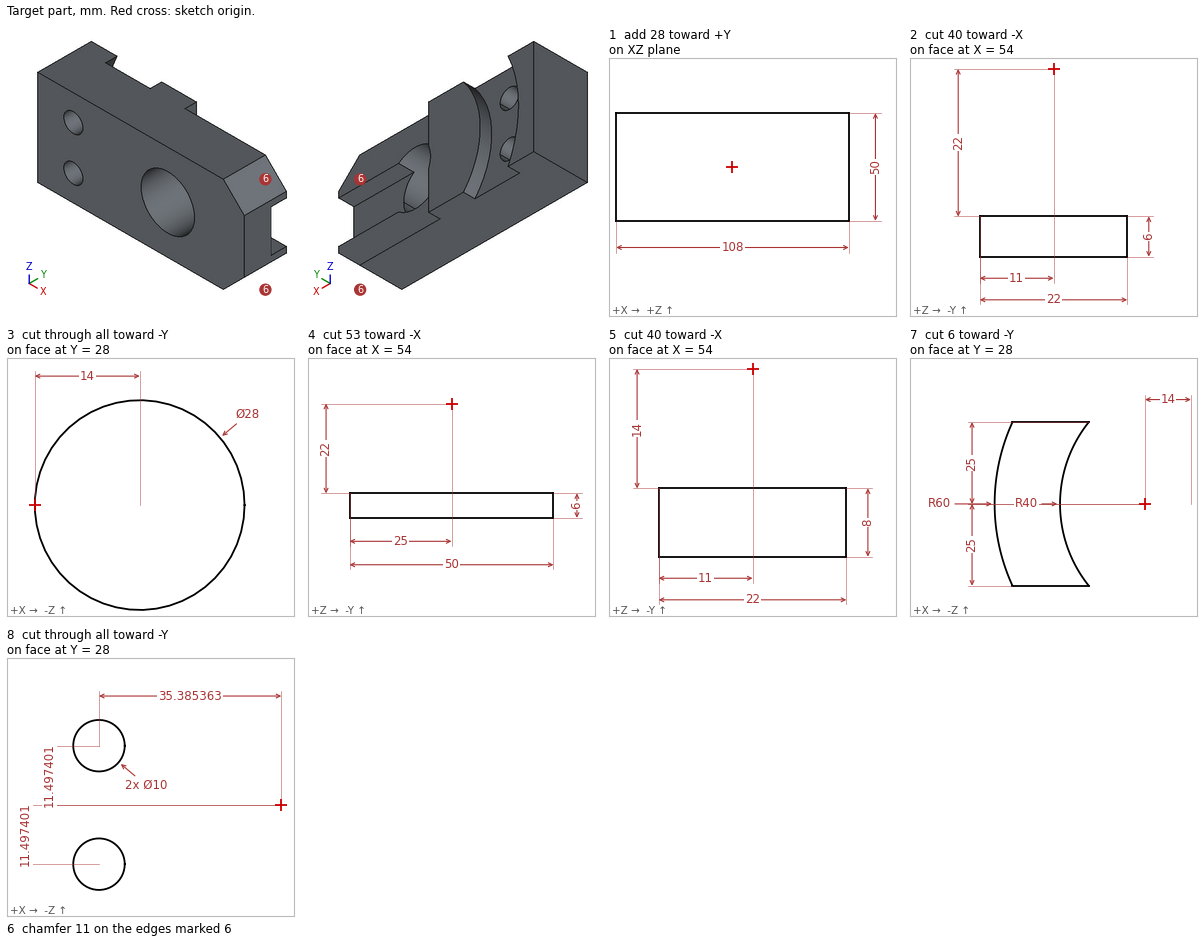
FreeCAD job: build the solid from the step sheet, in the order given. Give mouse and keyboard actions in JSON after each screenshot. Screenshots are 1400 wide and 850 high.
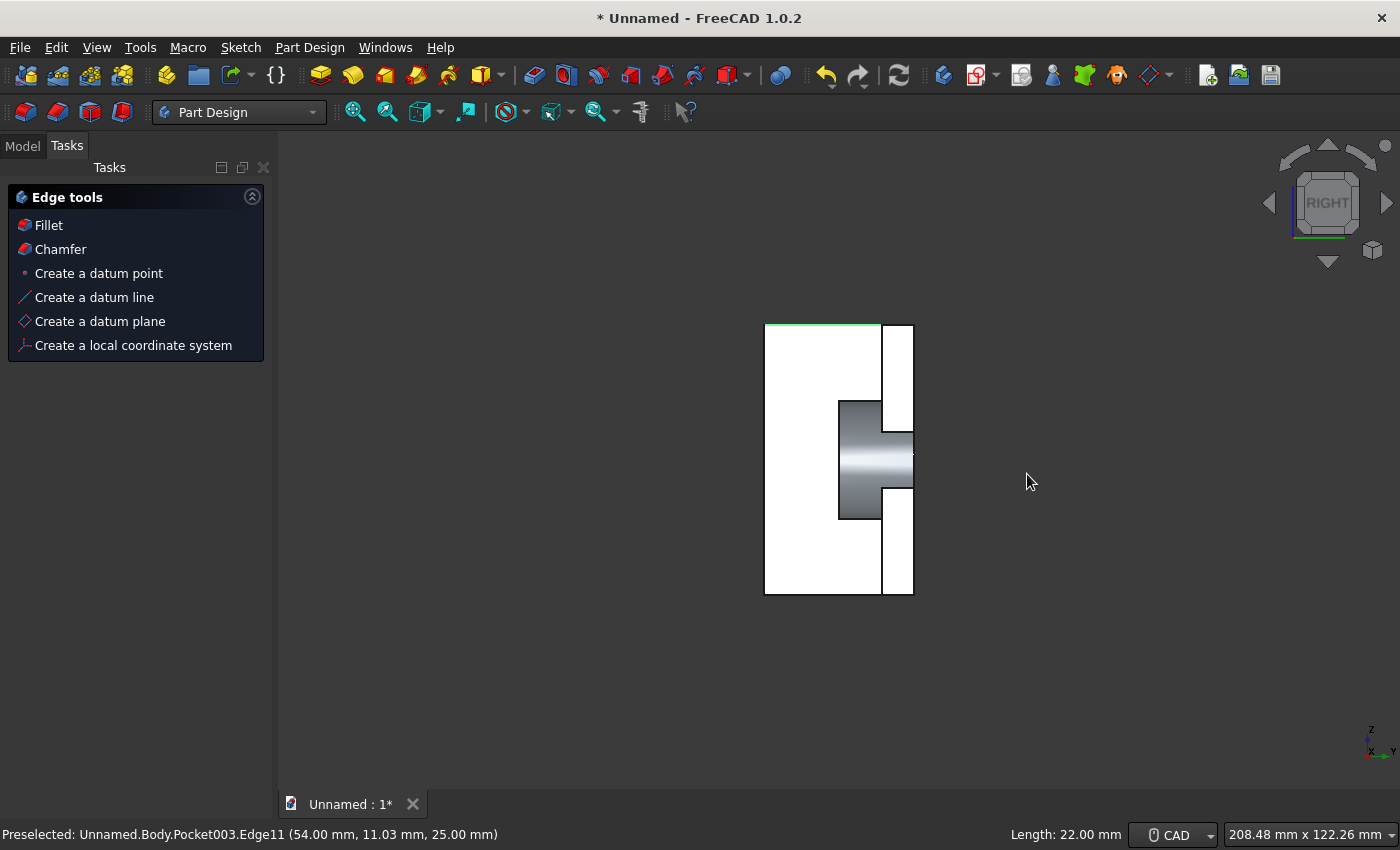
{"action": "key", "text": "v f"}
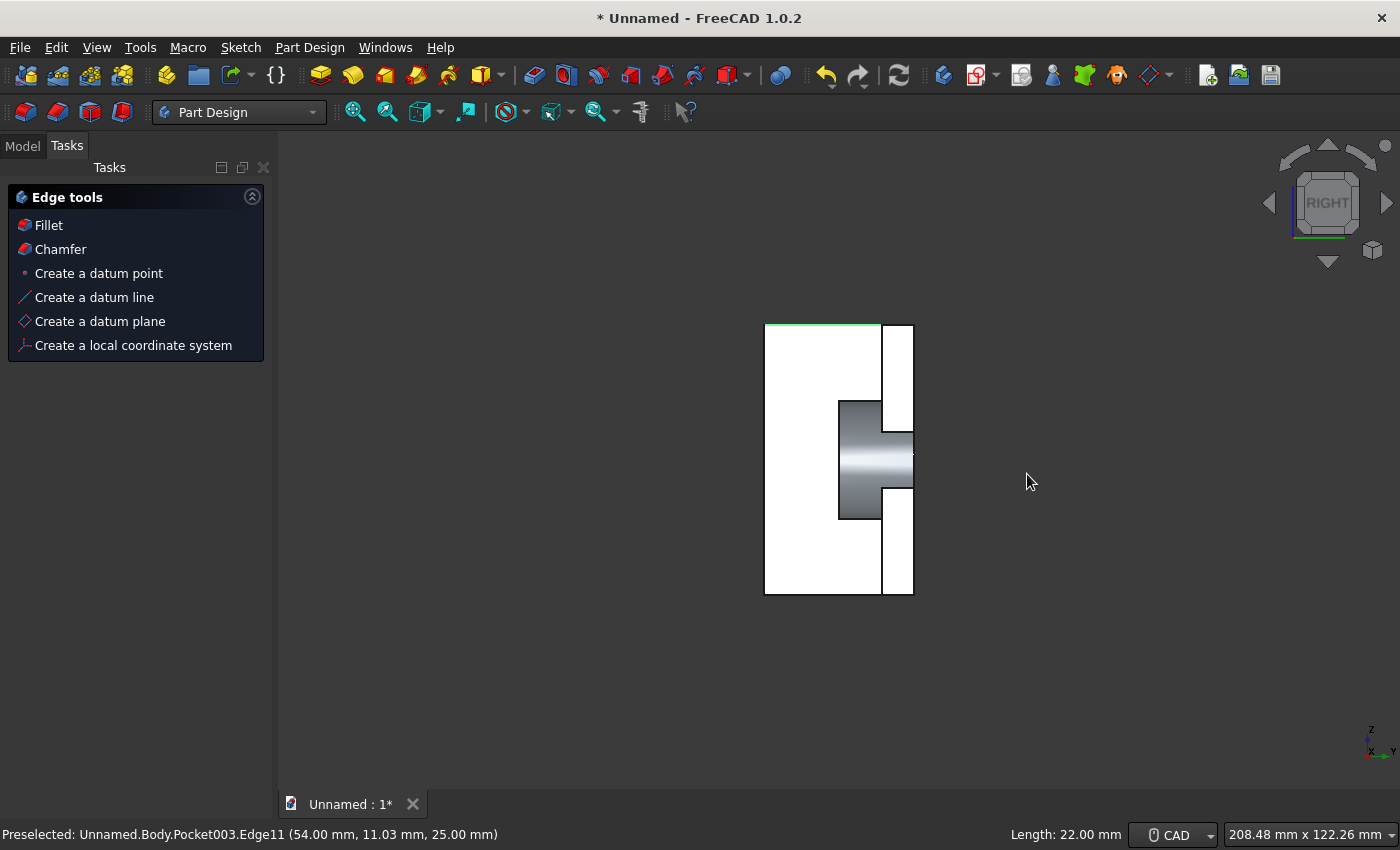
{"action": "left_click", "coordinate": [823, 594], "text": "ctrl"}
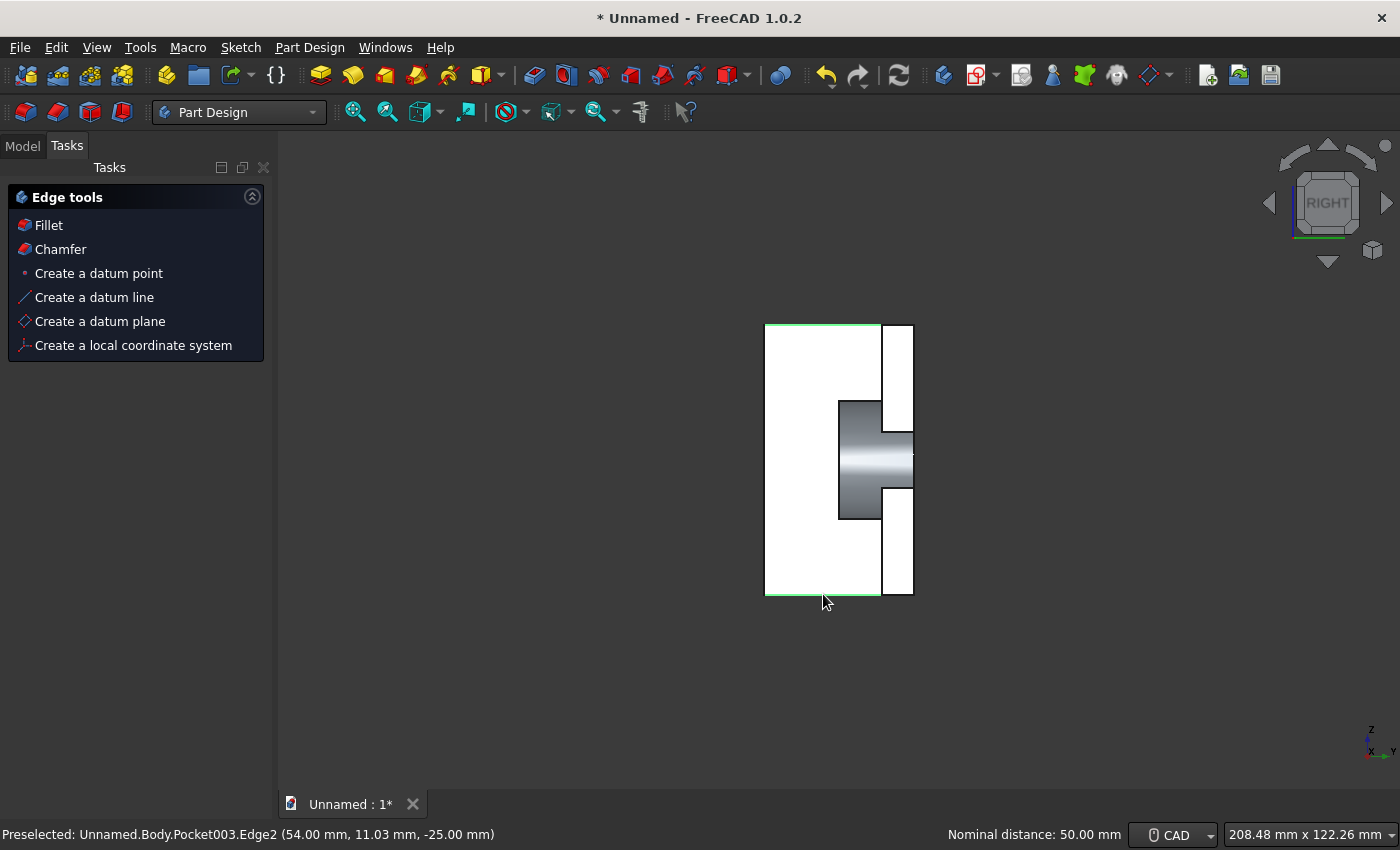
{"action": "left_click", "coordinate": [58, 112]}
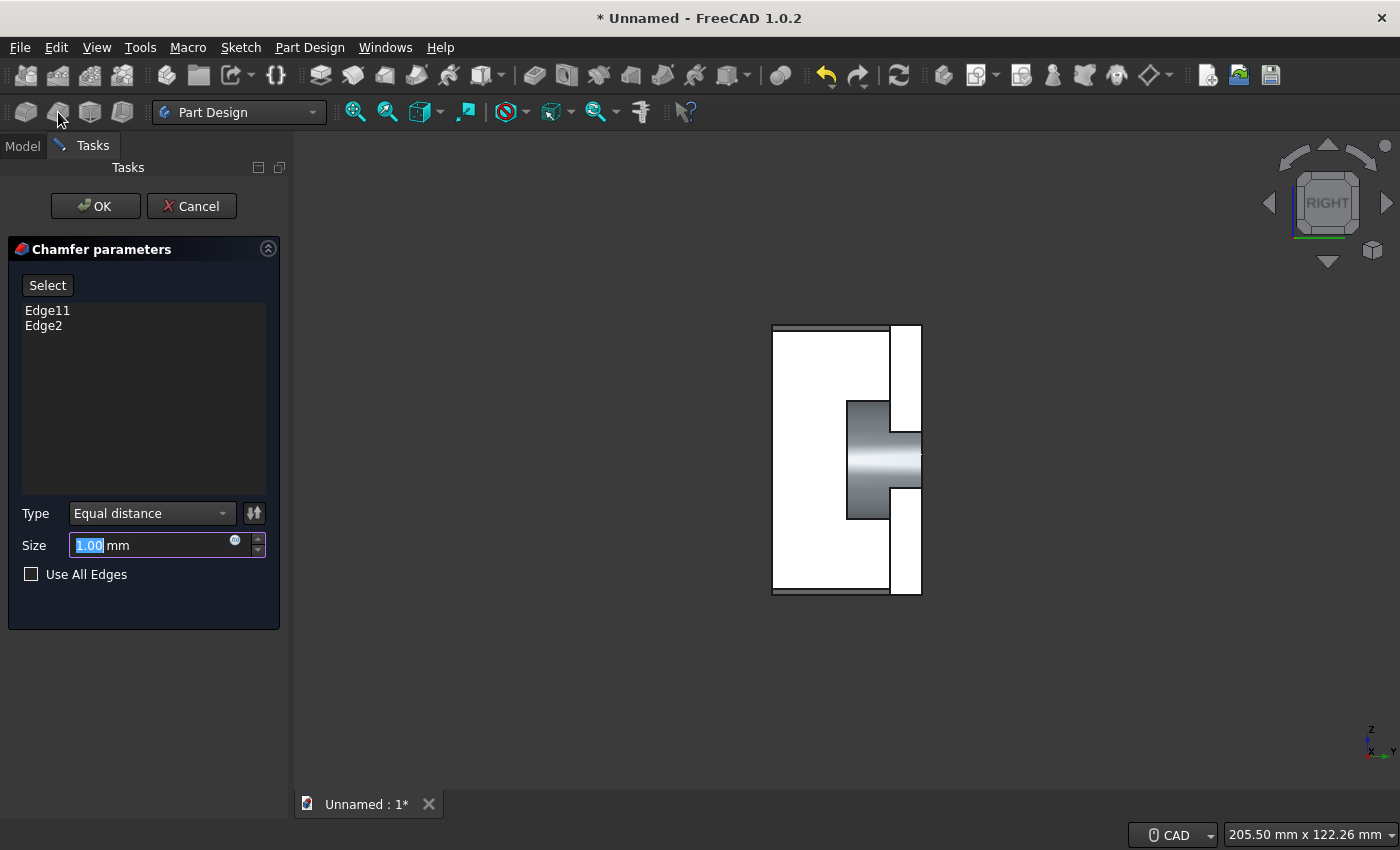
{"action": "type", "text": "11"}
{"action": "key", "text": "Tab"}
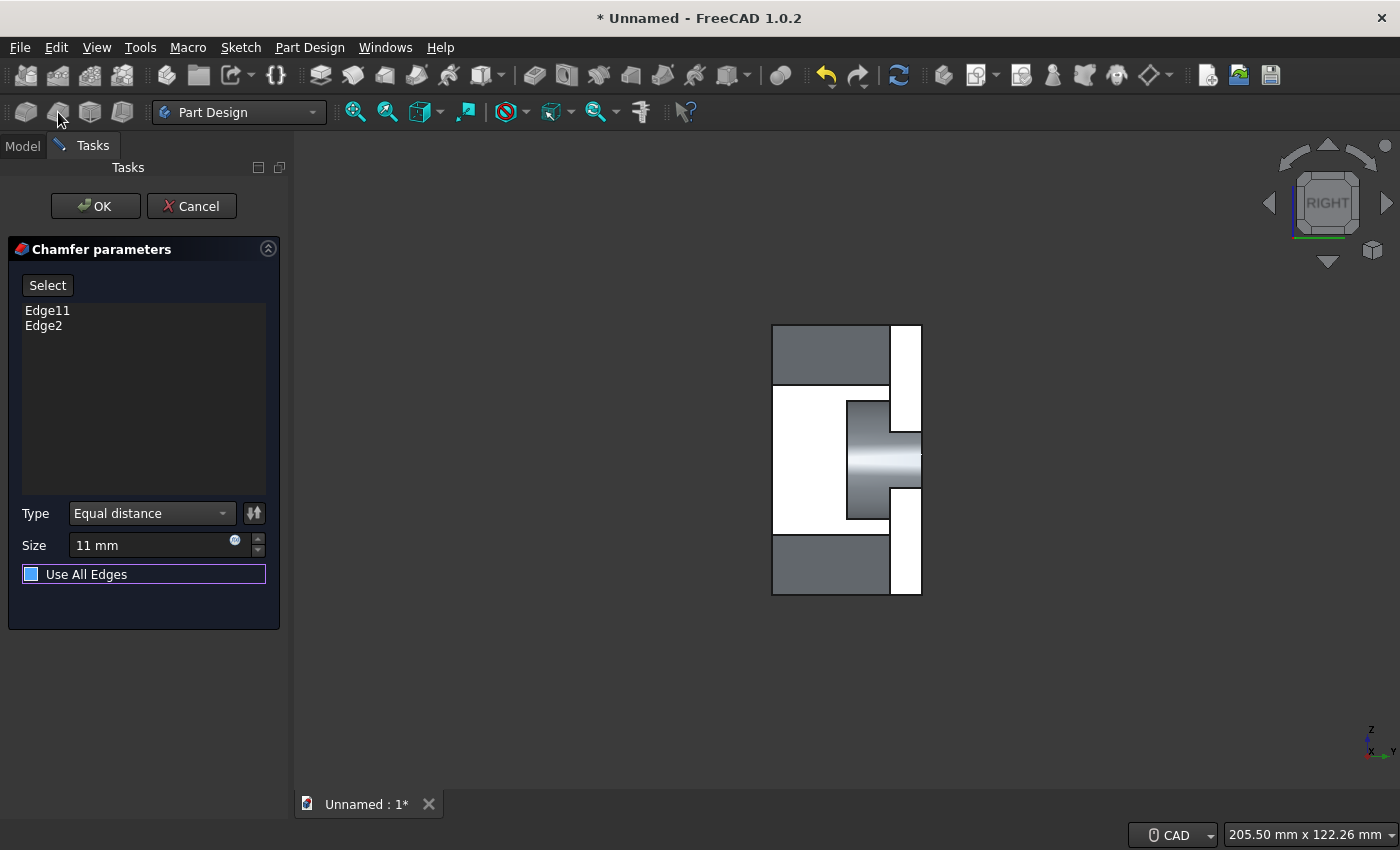
{"action": "left_click", "coordinate": [96, 206]}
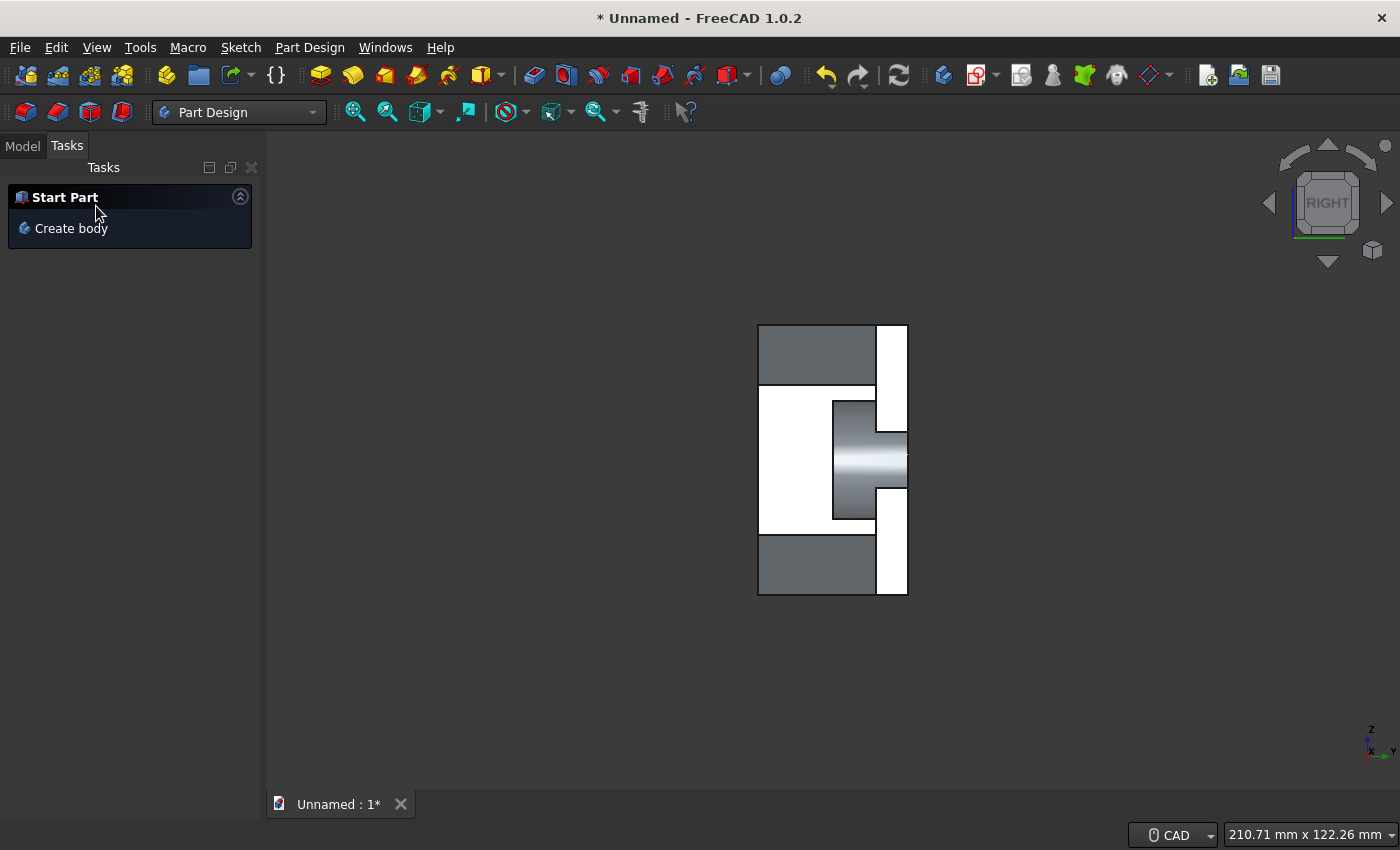
{"action": "key", "text": "v f"}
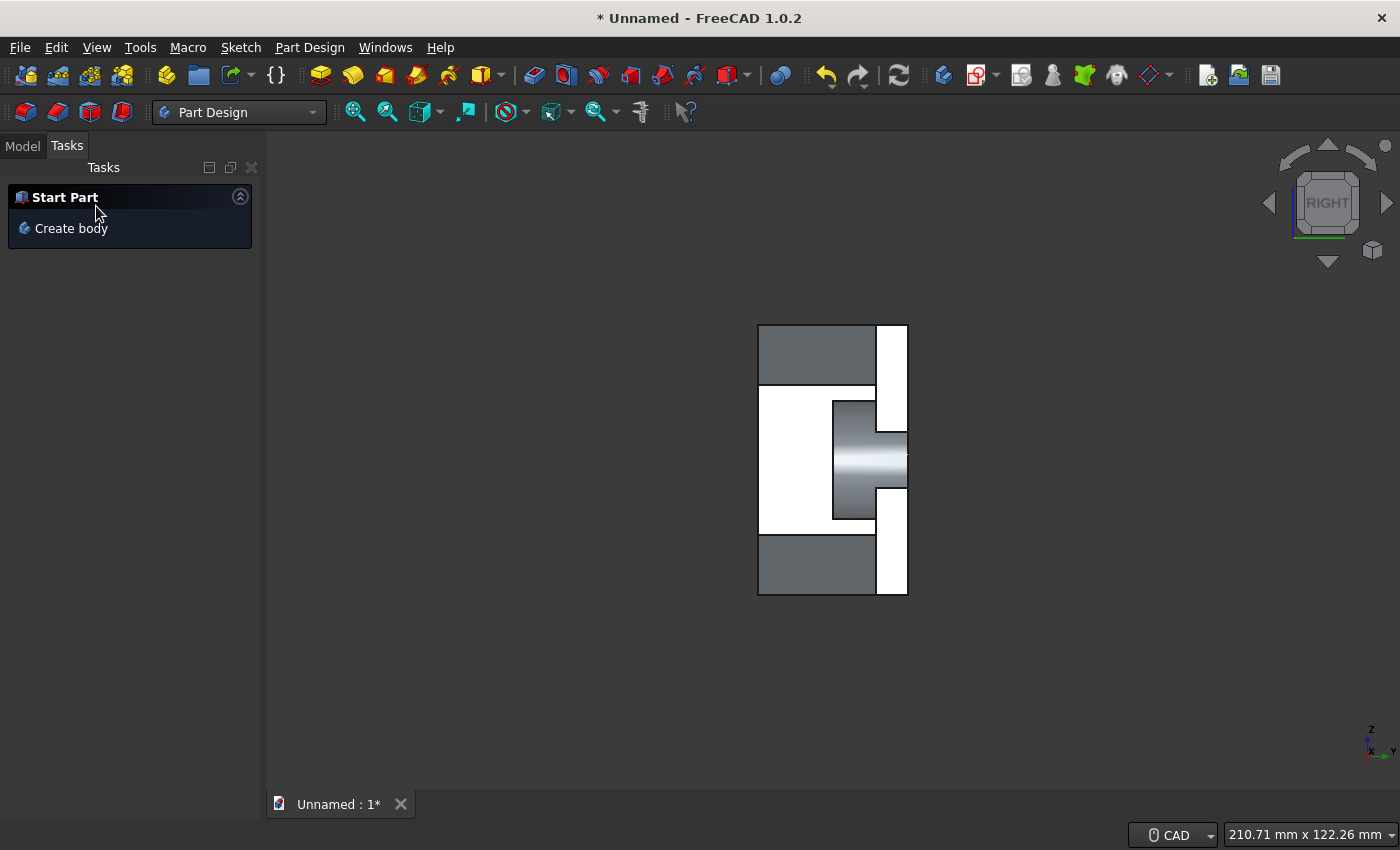
{"action": "key", "text": "4"}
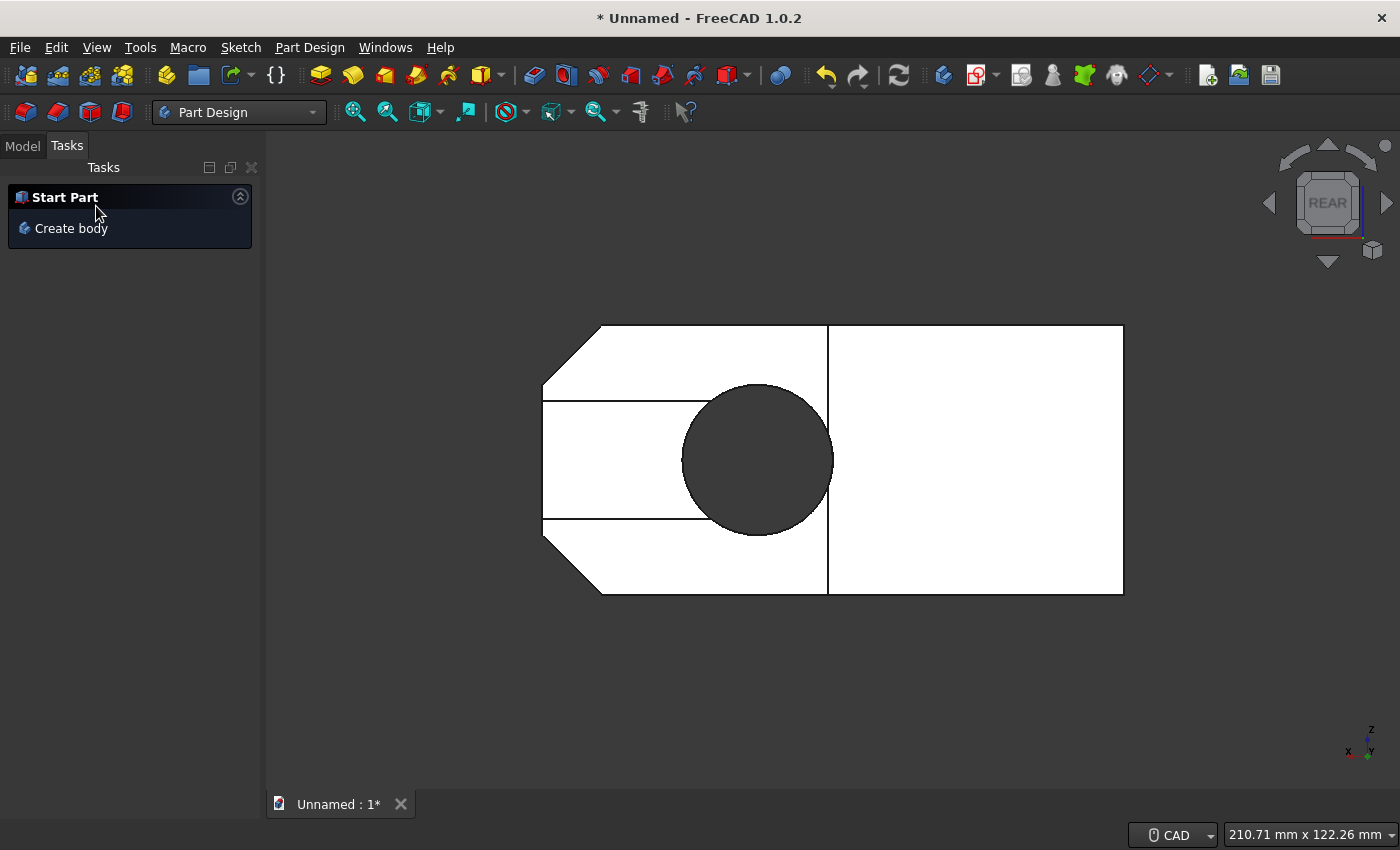
{"action": "left_click", "coordinate": [976, 459]}